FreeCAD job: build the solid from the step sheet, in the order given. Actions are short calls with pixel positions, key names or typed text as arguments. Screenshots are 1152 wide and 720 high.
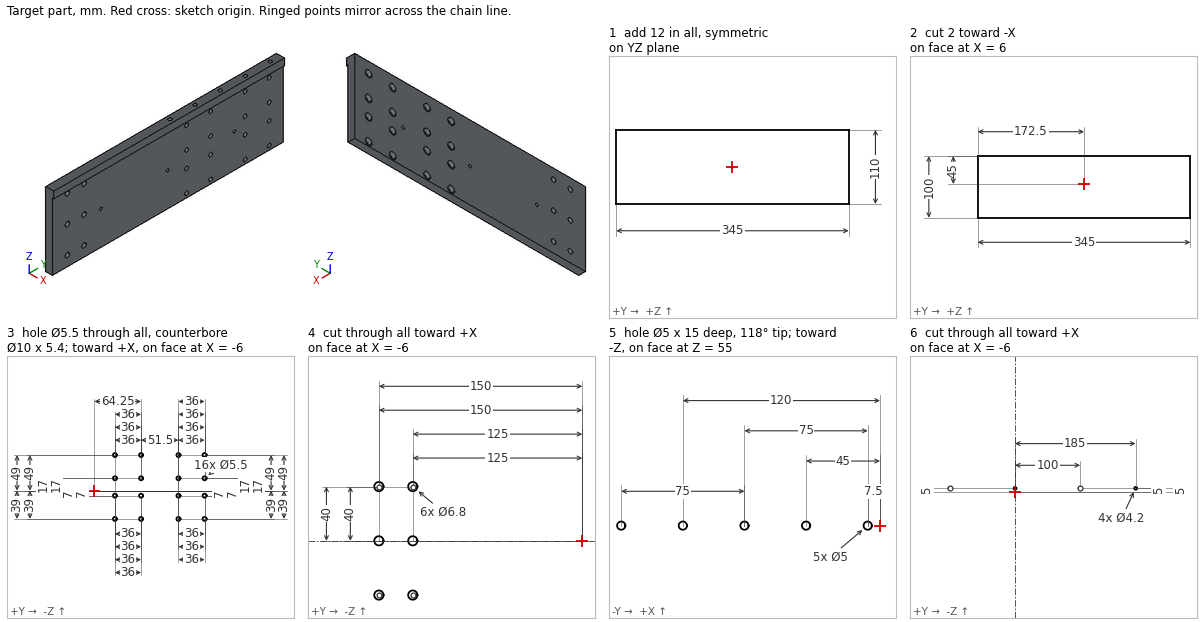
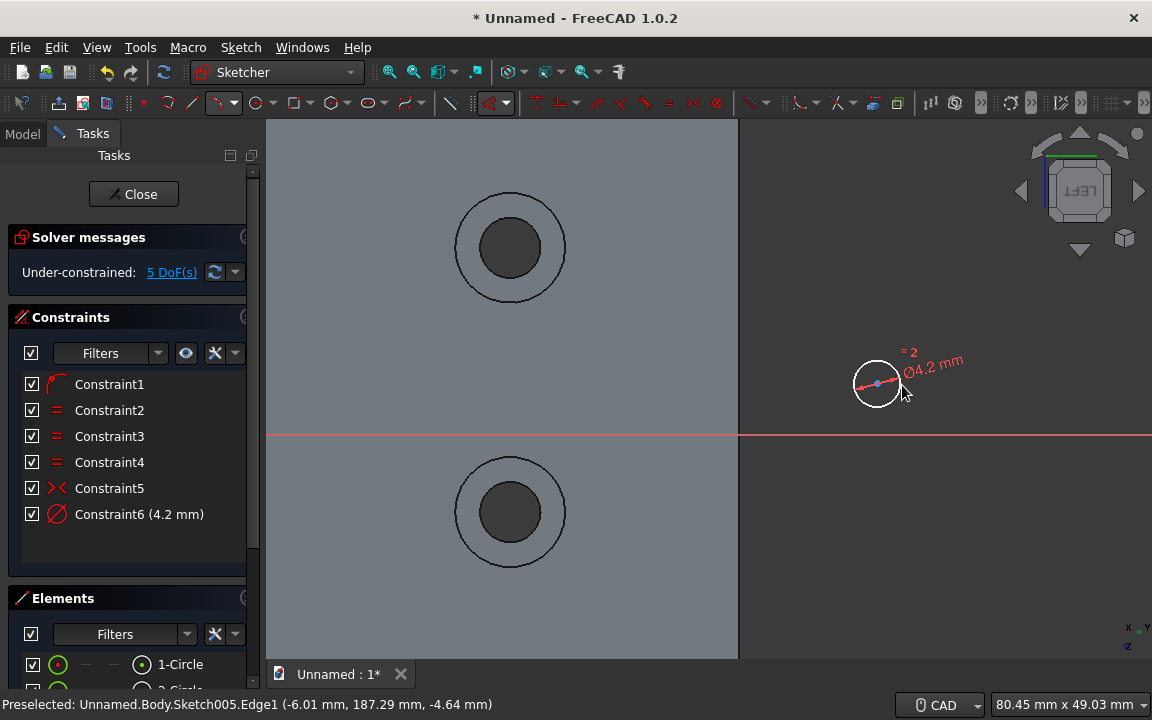
click(877, 384)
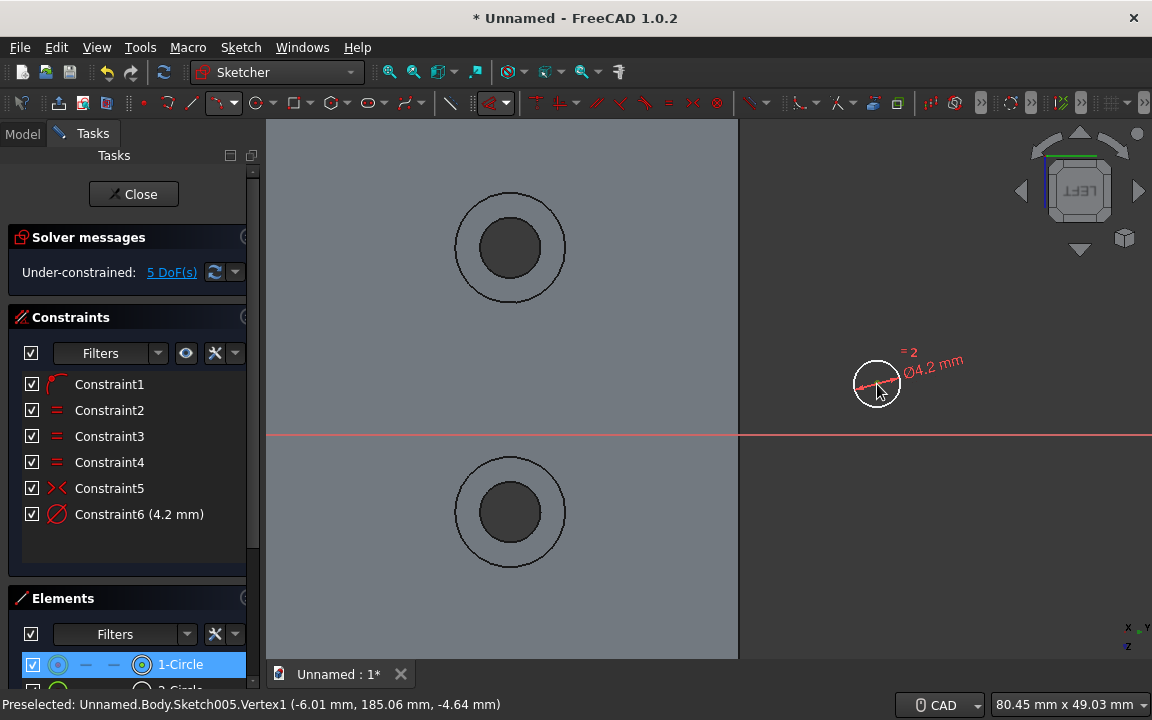
click(508, 104)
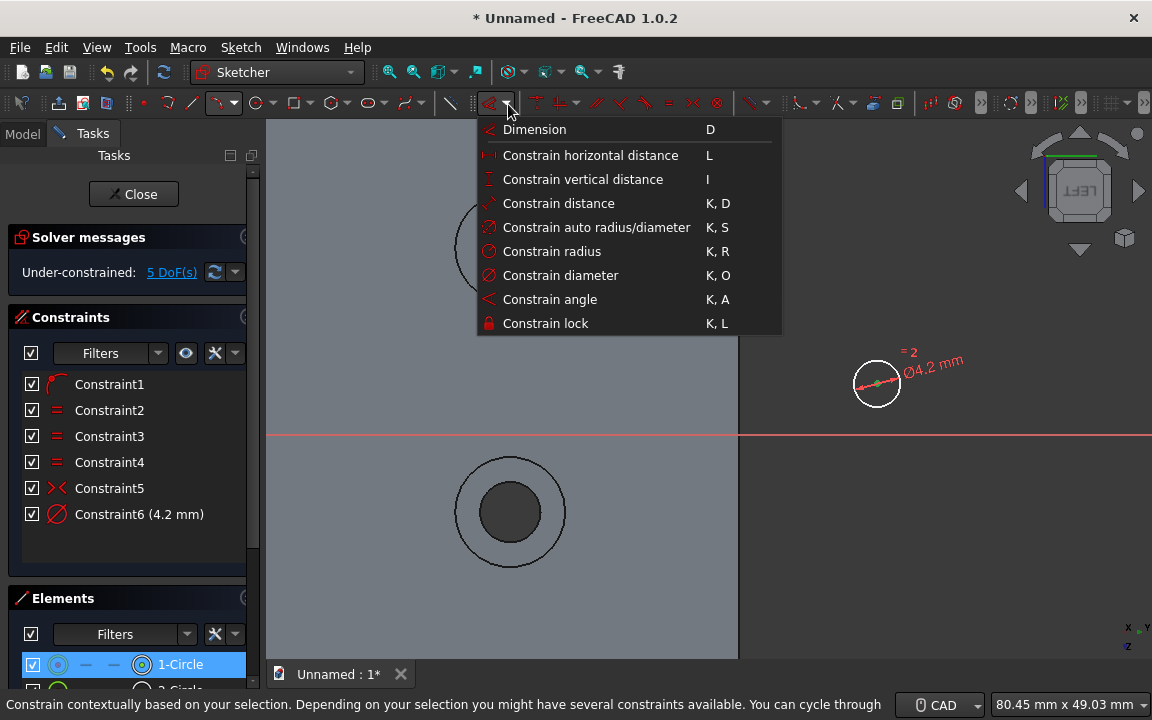
click(630, 179)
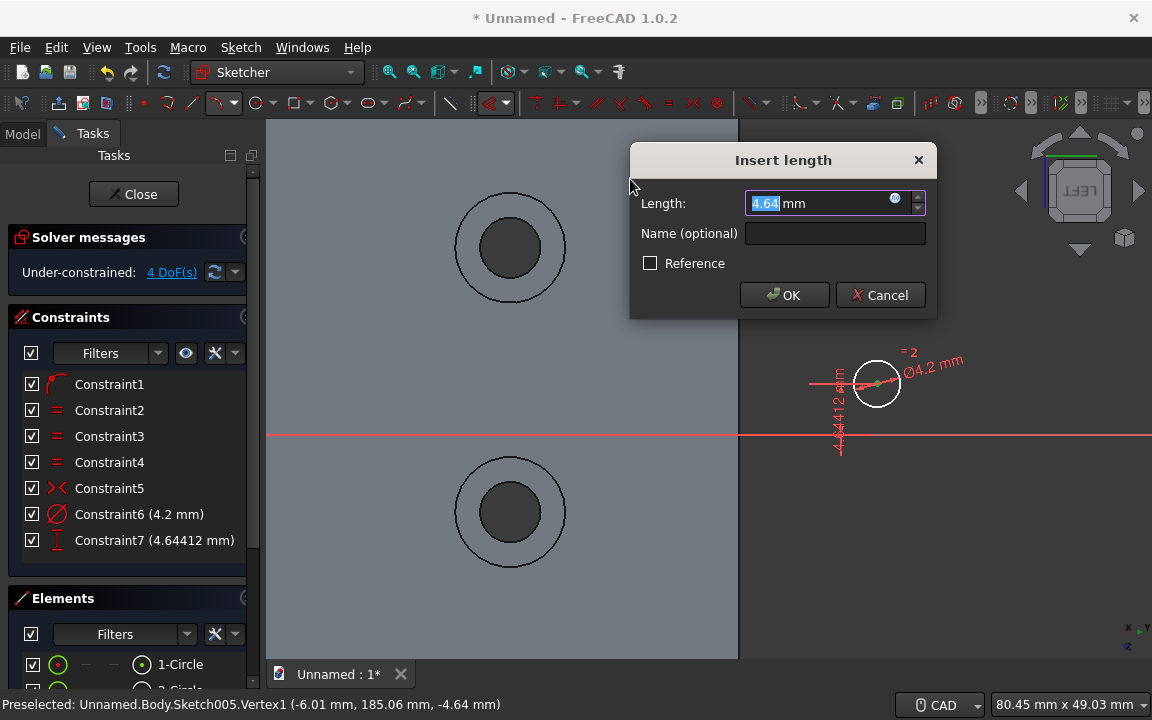
text(5)
key(Return)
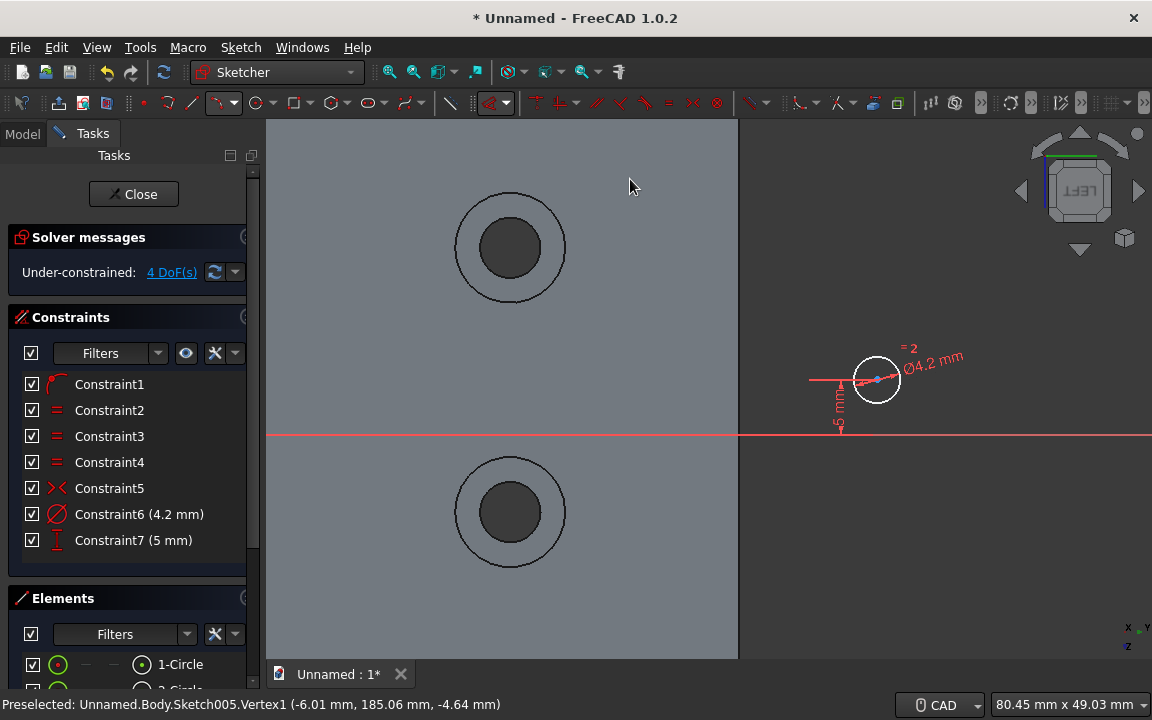
scroll(905, 388, down, 9)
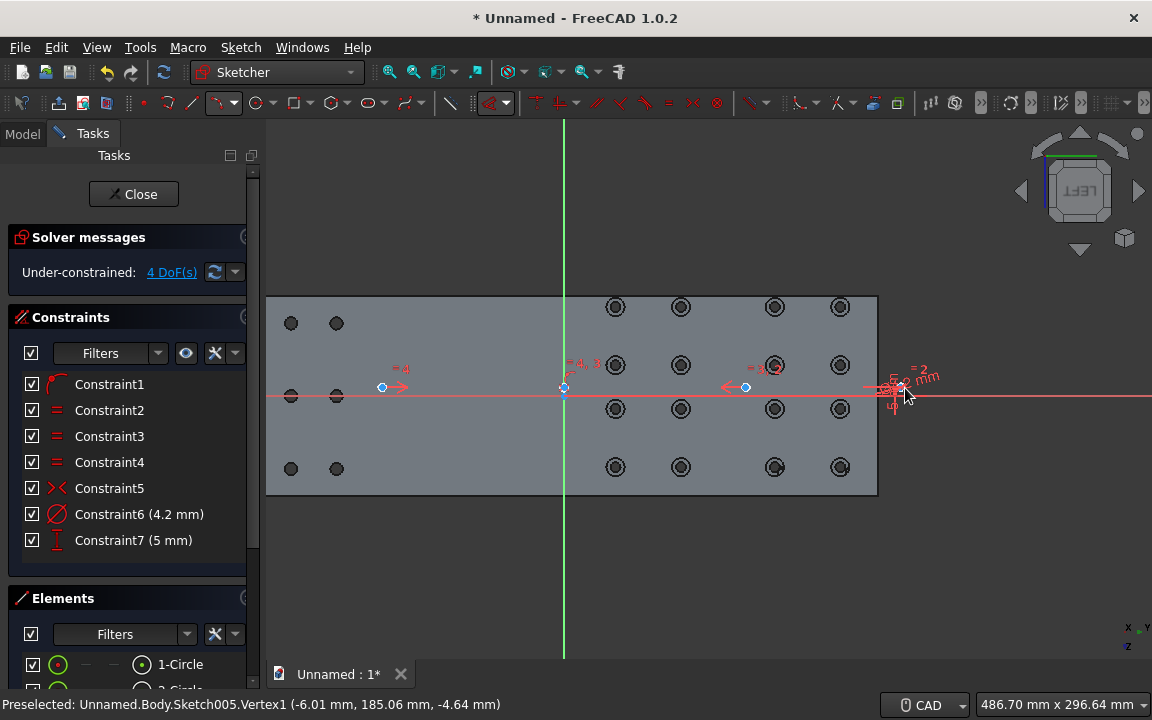
scroll(746, 387, up, 8)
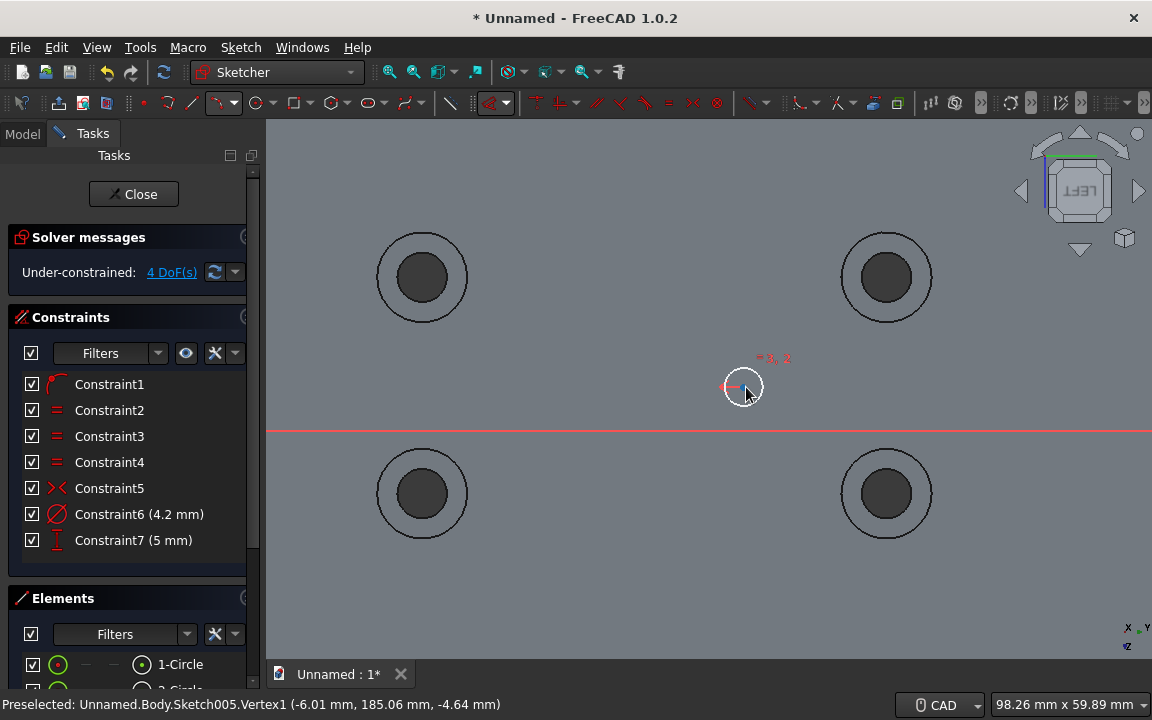
click(744, 387)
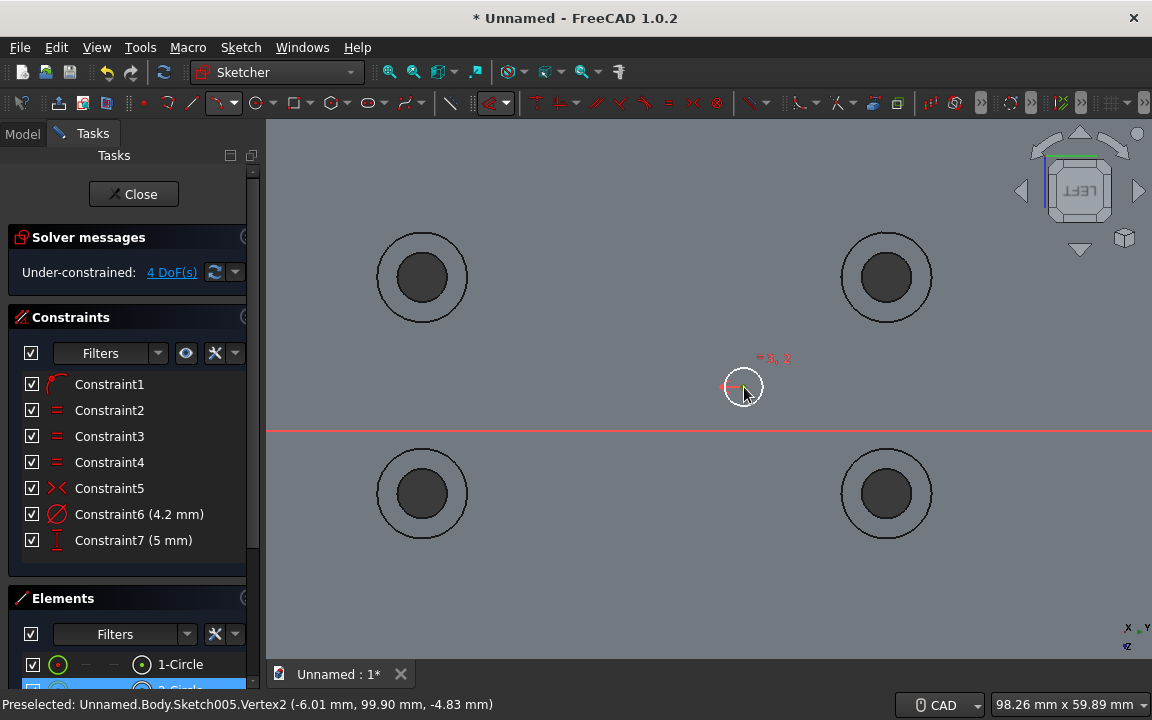
click(508, 104)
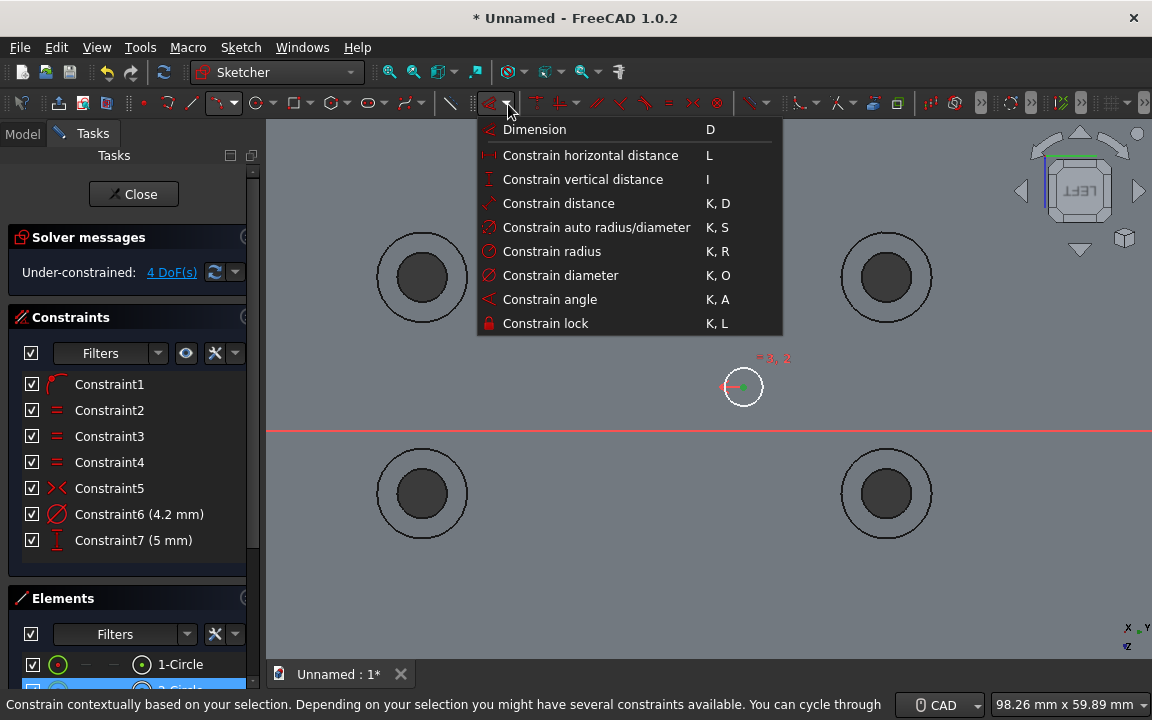
click(630, 179)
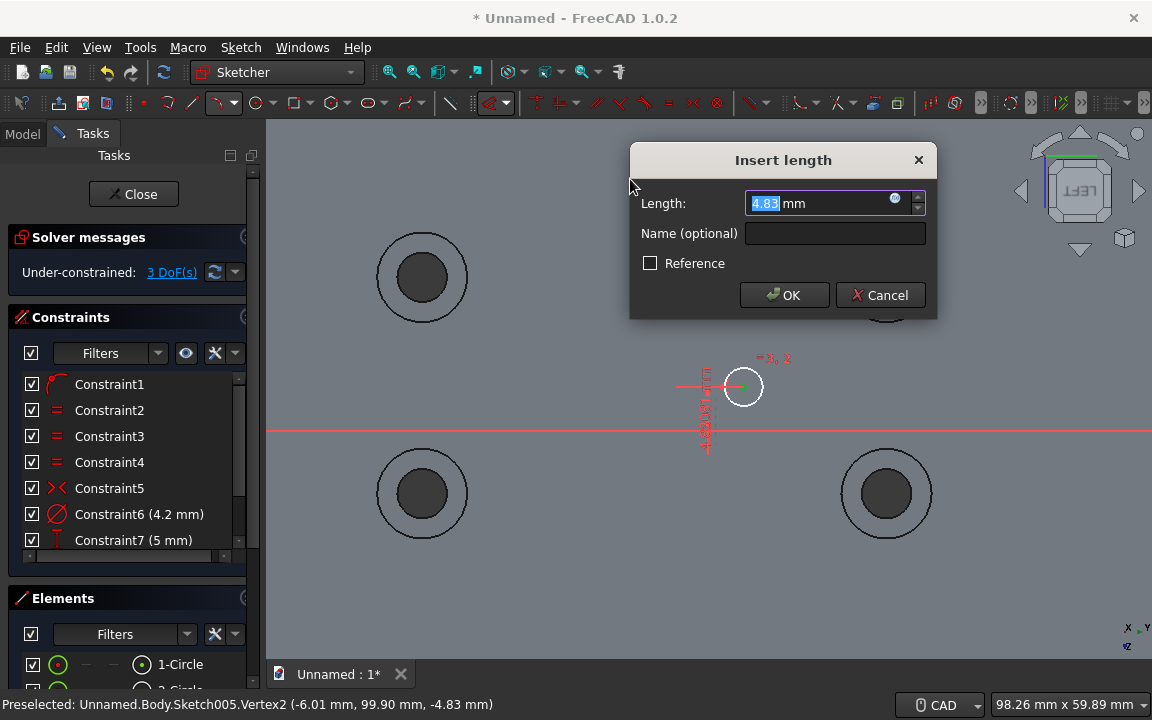
text(5)
key(Return)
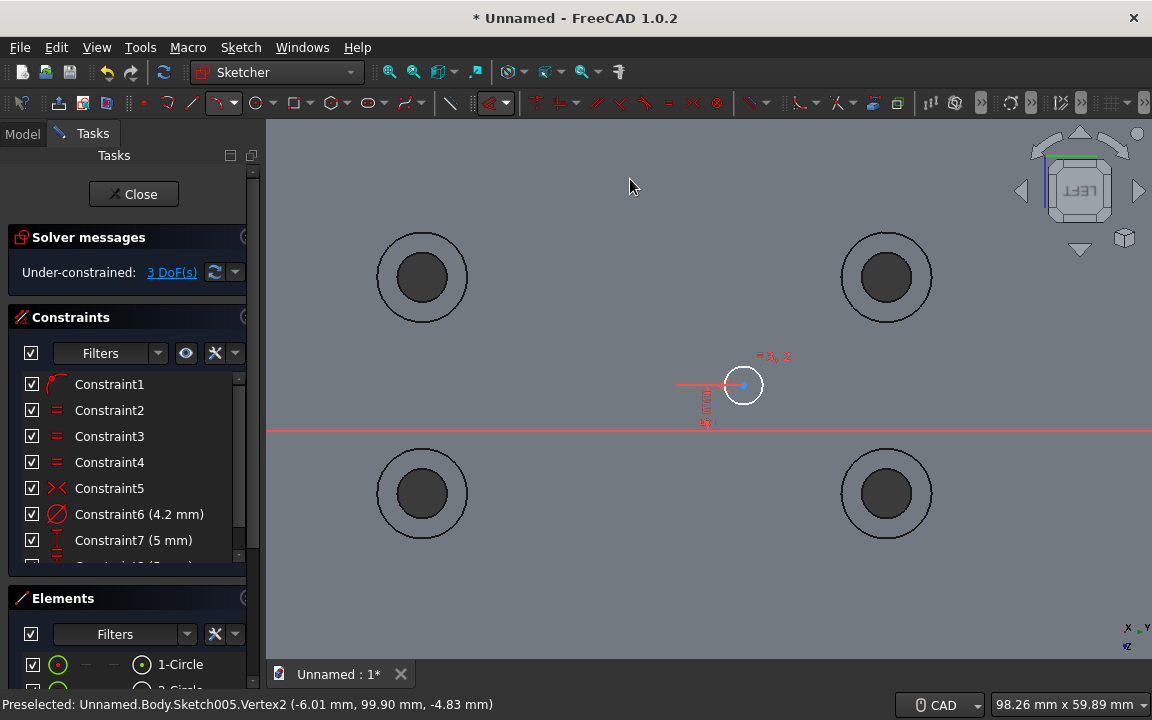
scroll(745, 387, down, 8)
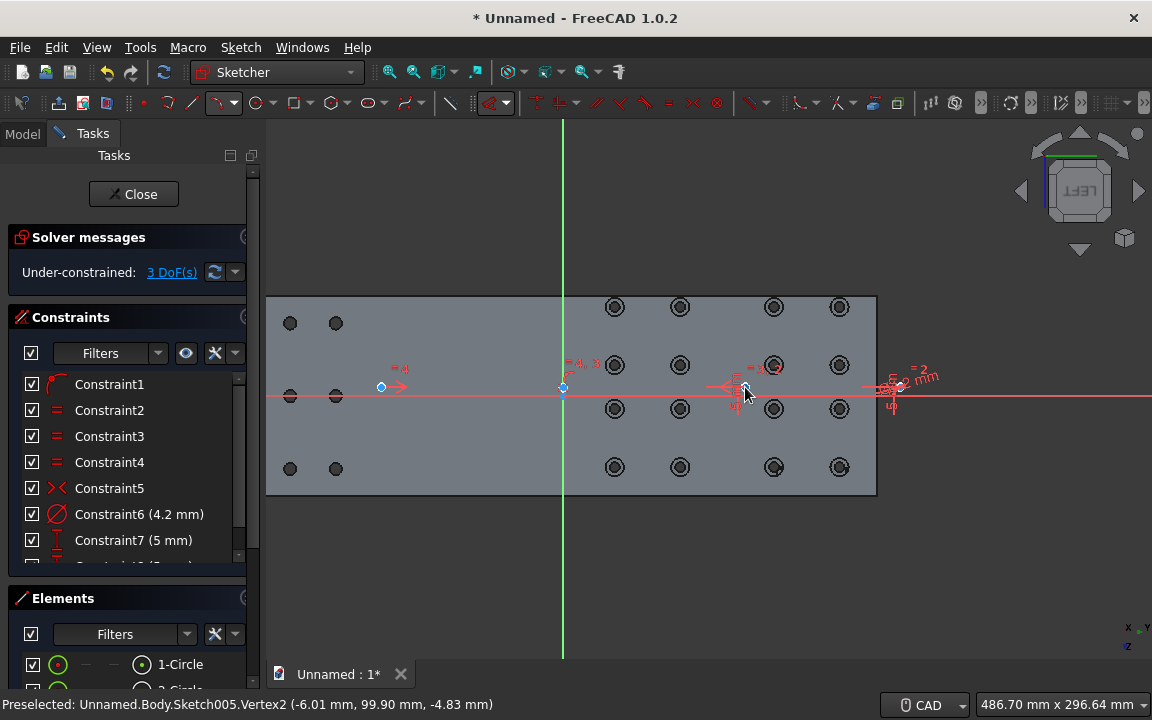
scroll(563, 388, up, 8)